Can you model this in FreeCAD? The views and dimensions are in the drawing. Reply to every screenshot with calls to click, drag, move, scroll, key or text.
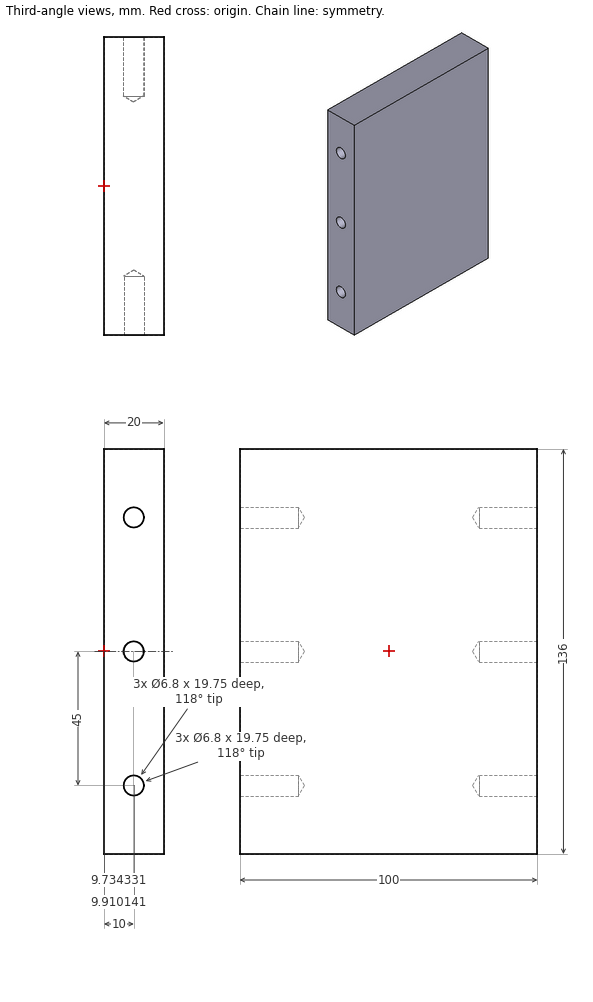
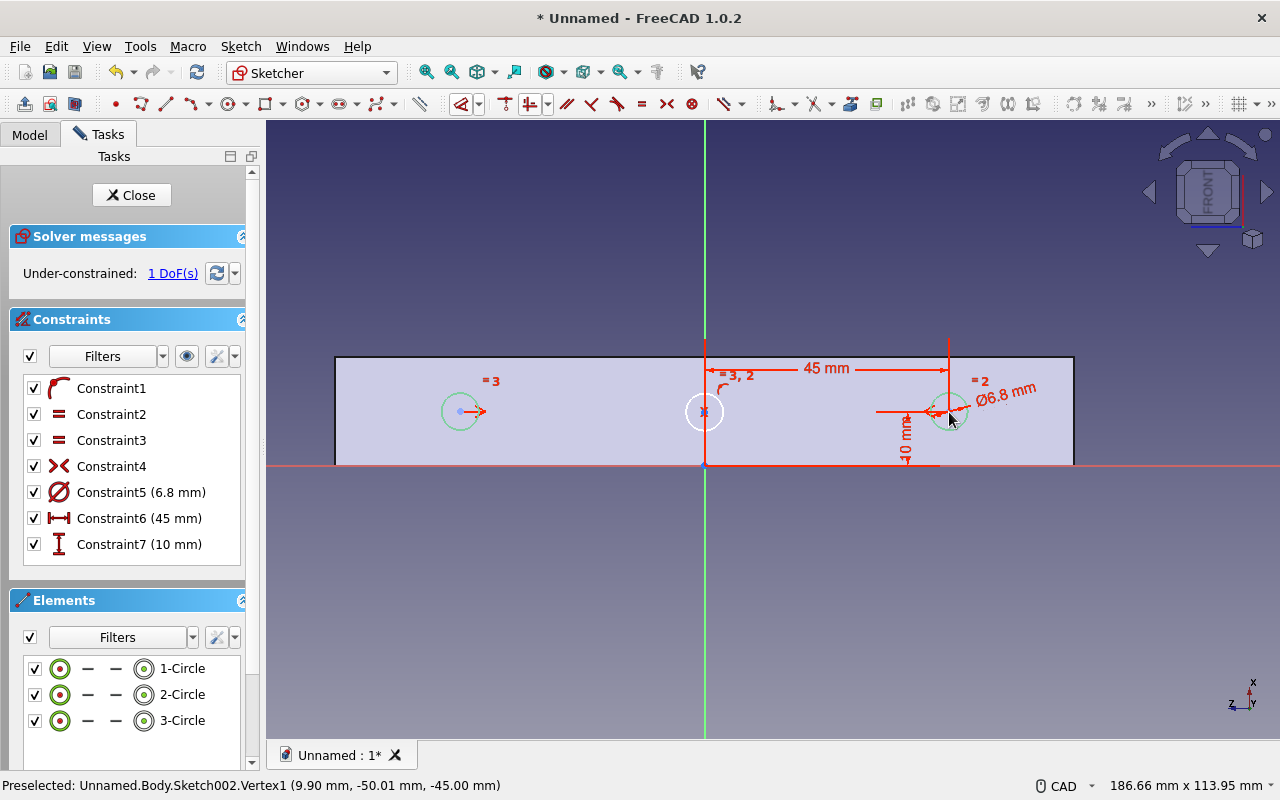
click(705, 412)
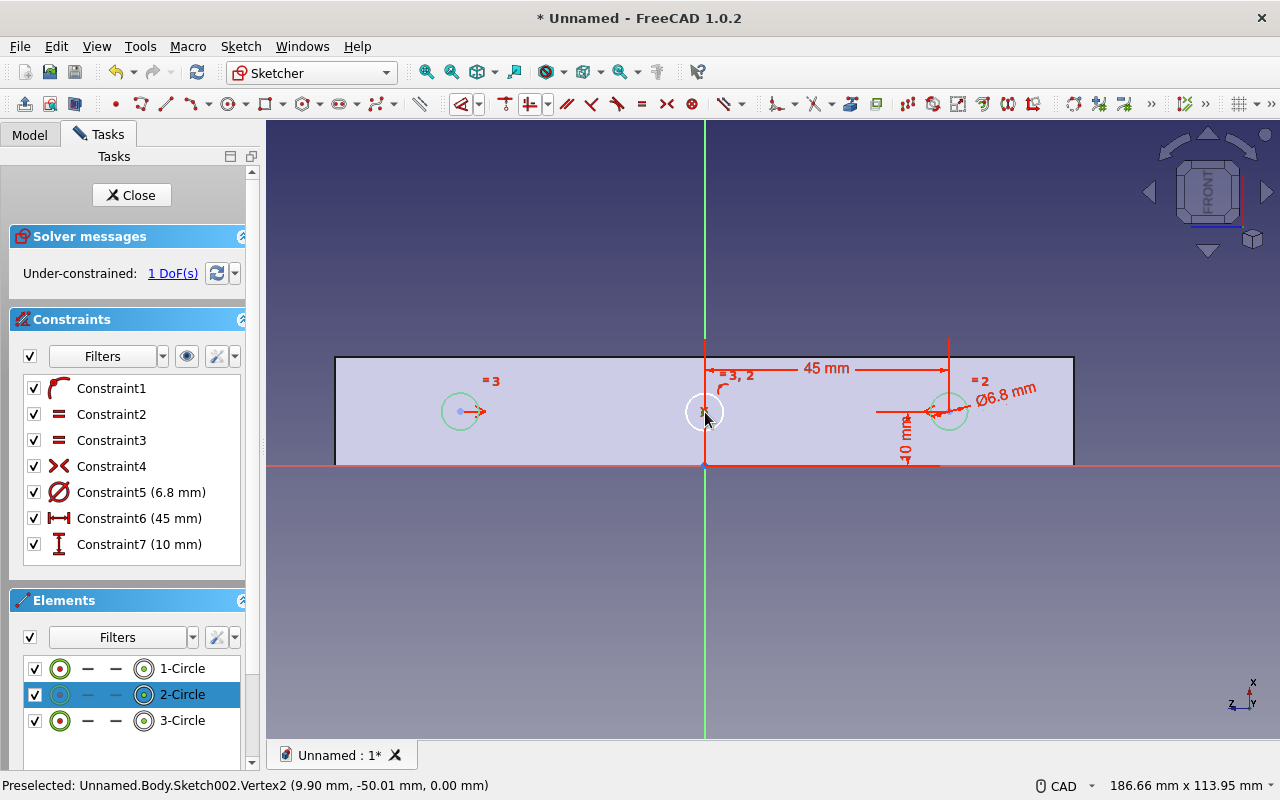
click(478, 104)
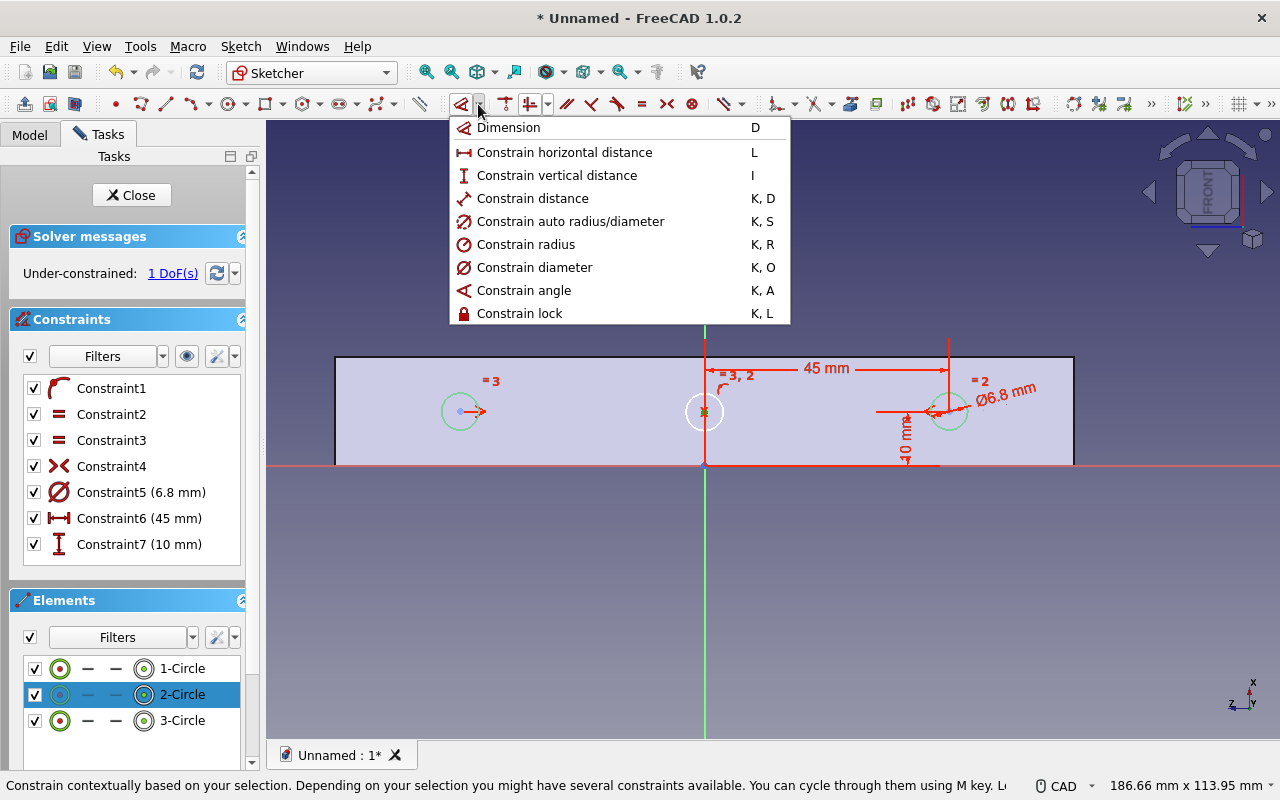
click(620, 176)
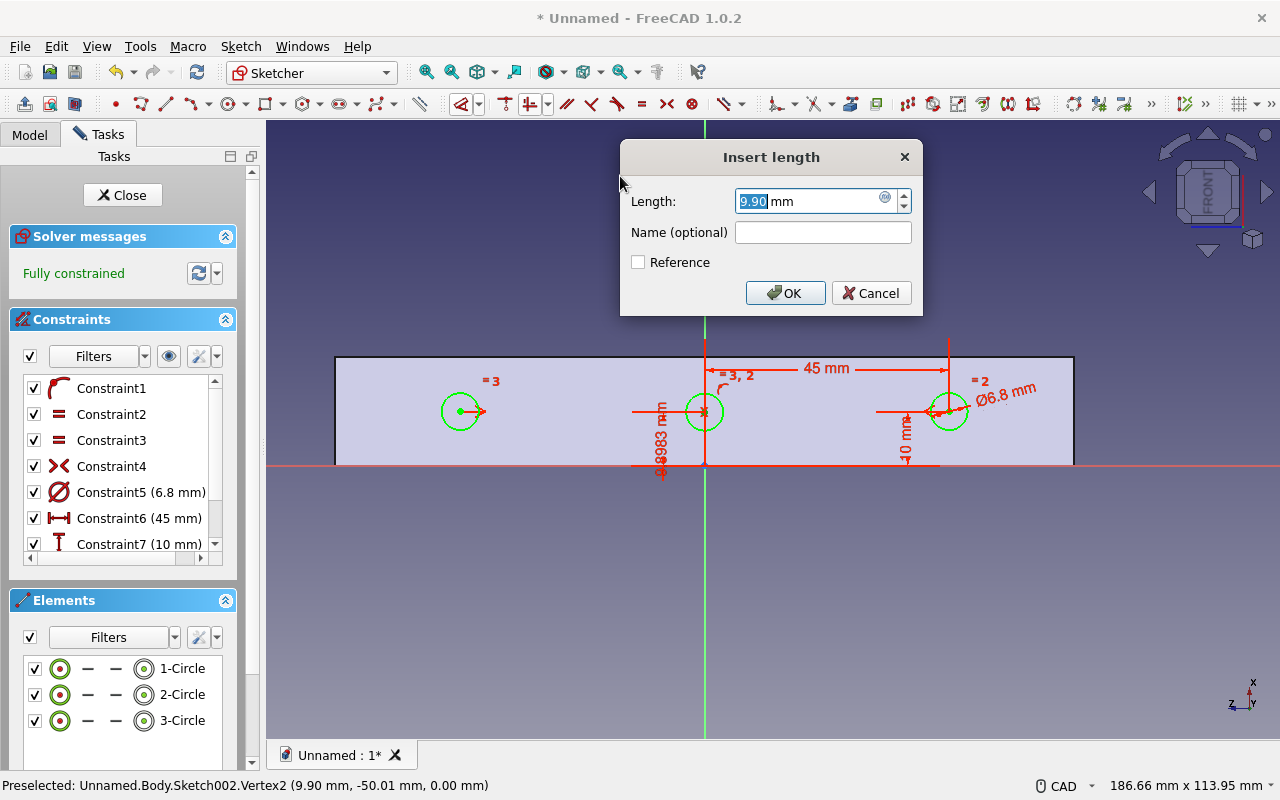
text(10)
key(Return)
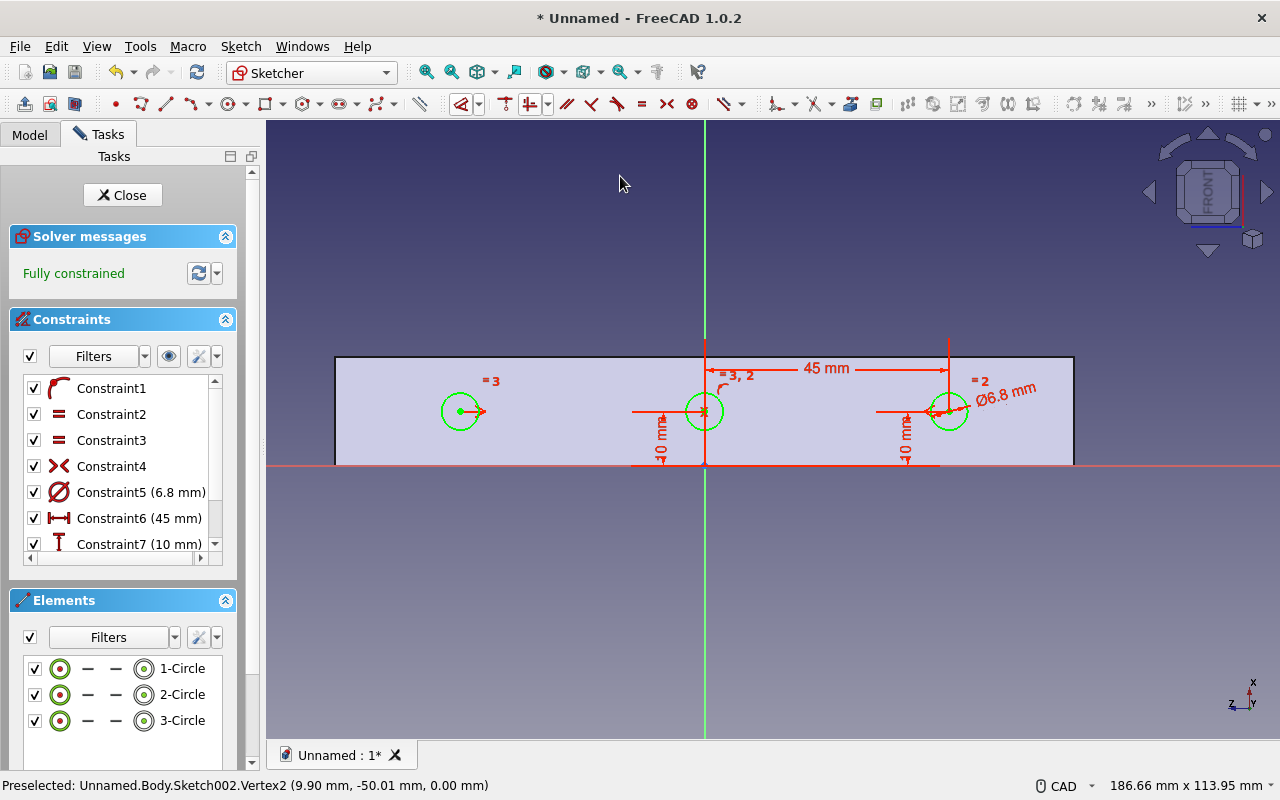
click(123, 195)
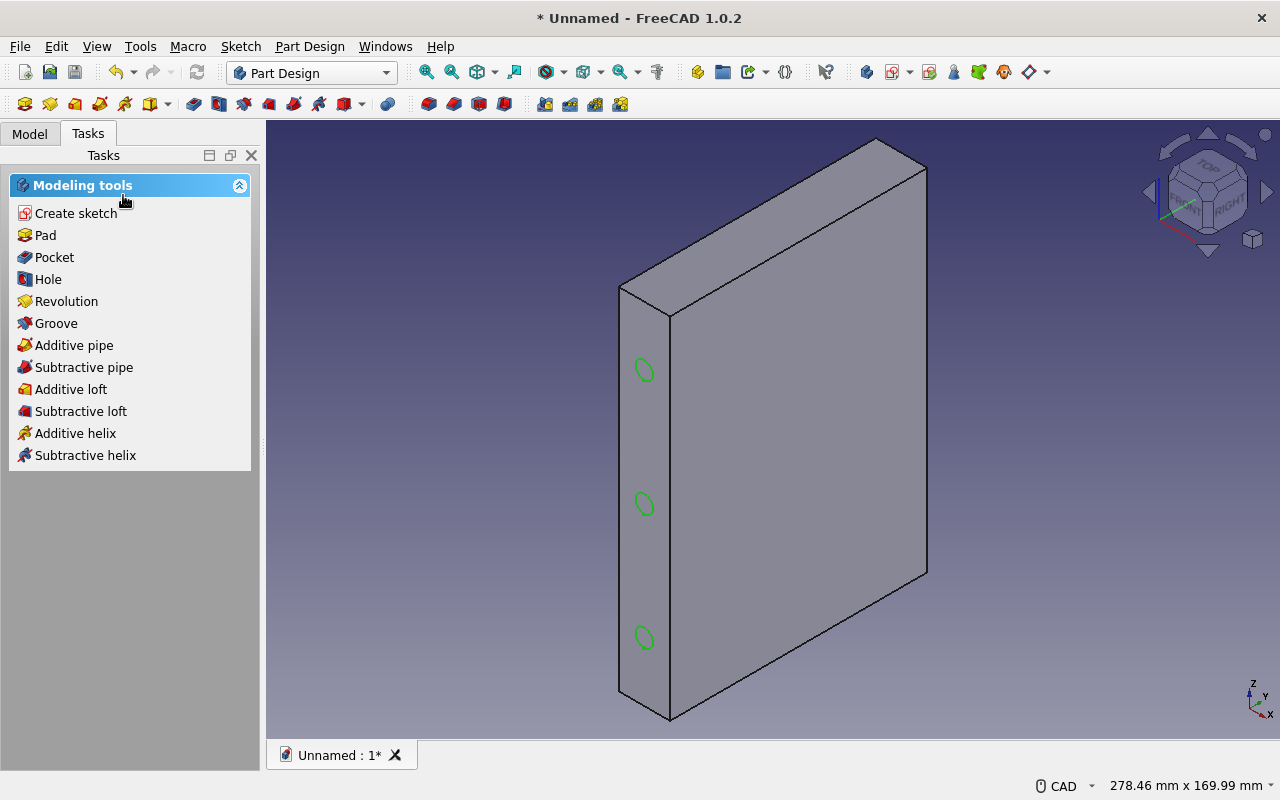
click(219, 104)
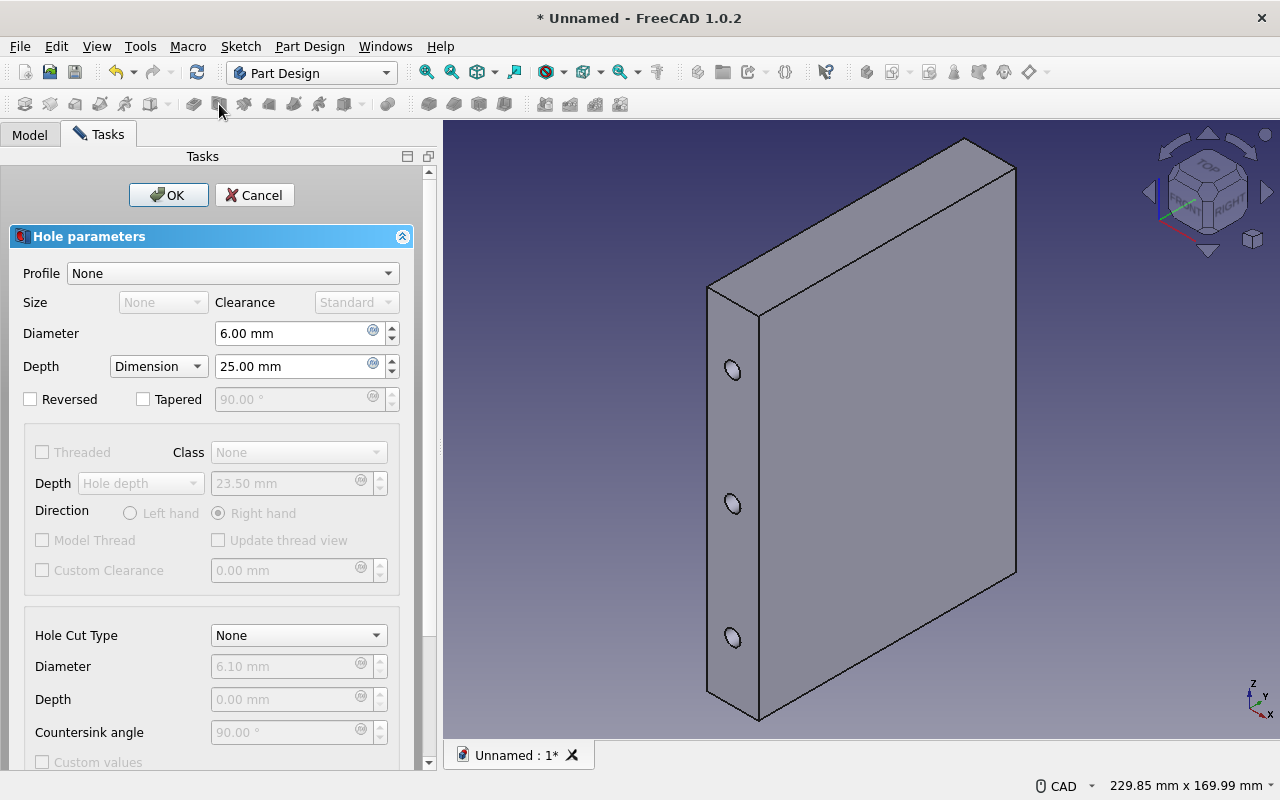
triple_click(300, 334)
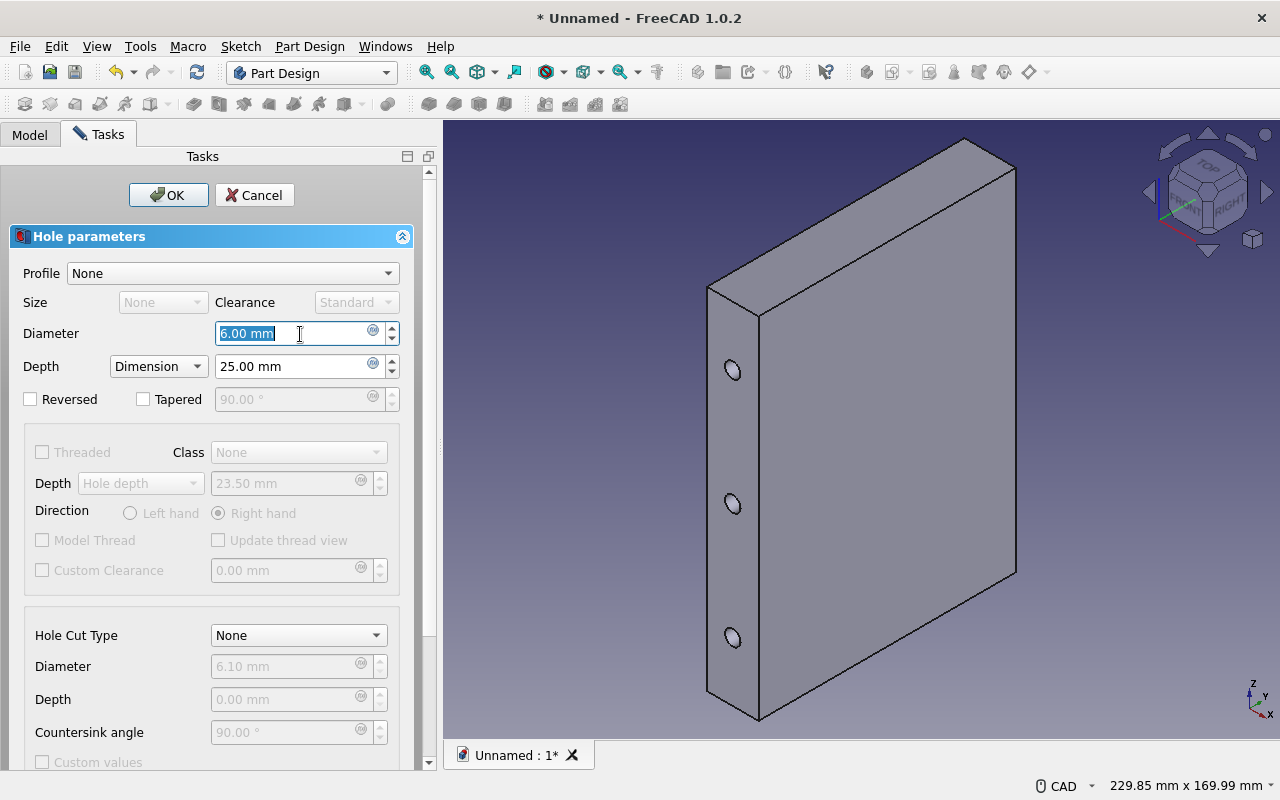
text(6.8)
key(Tab)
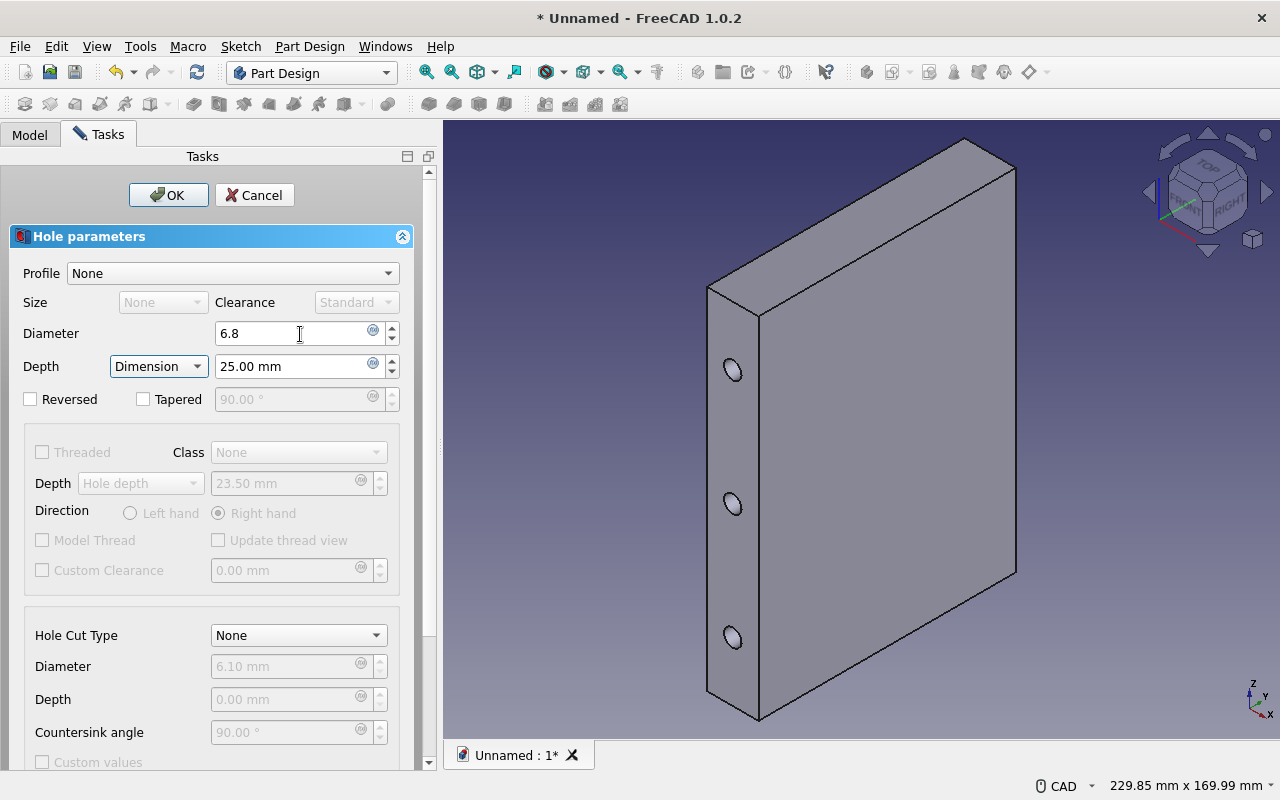
triple_click(300, 366)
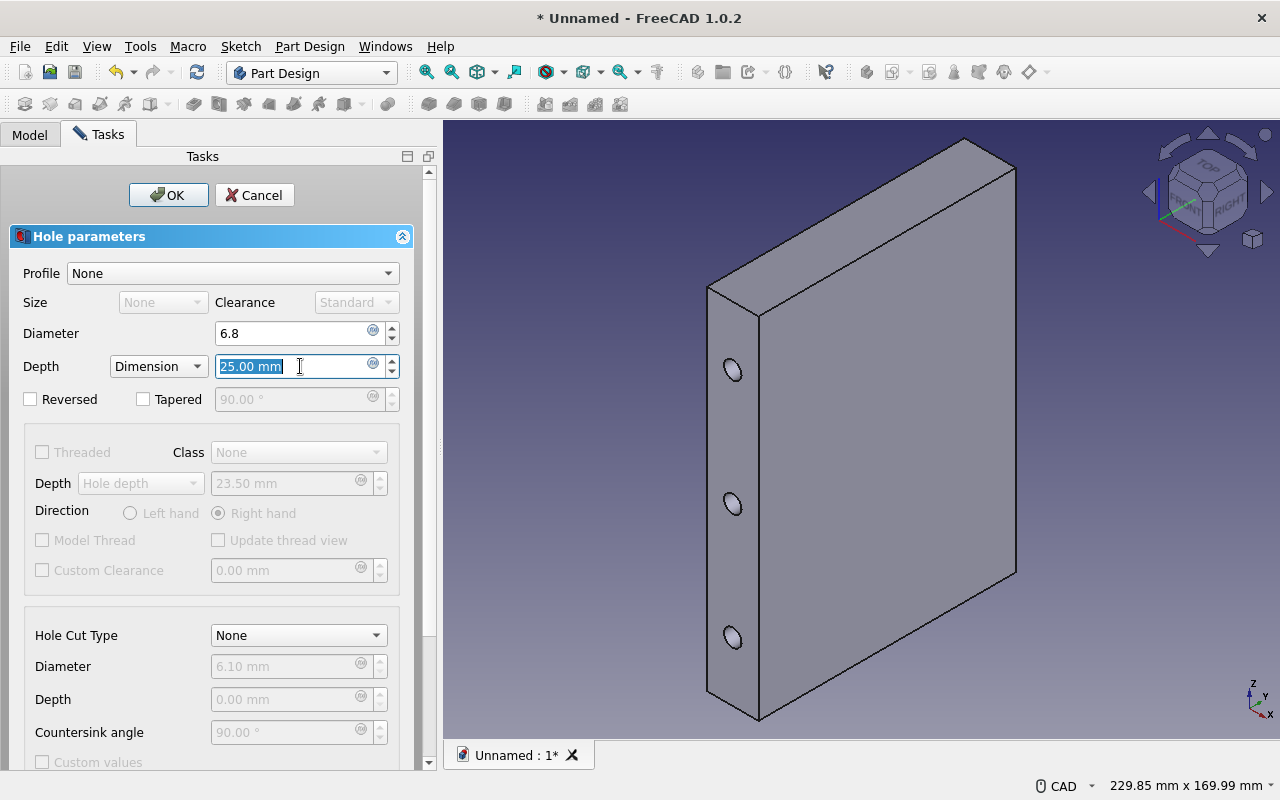
text(19.75)
key(Tab)